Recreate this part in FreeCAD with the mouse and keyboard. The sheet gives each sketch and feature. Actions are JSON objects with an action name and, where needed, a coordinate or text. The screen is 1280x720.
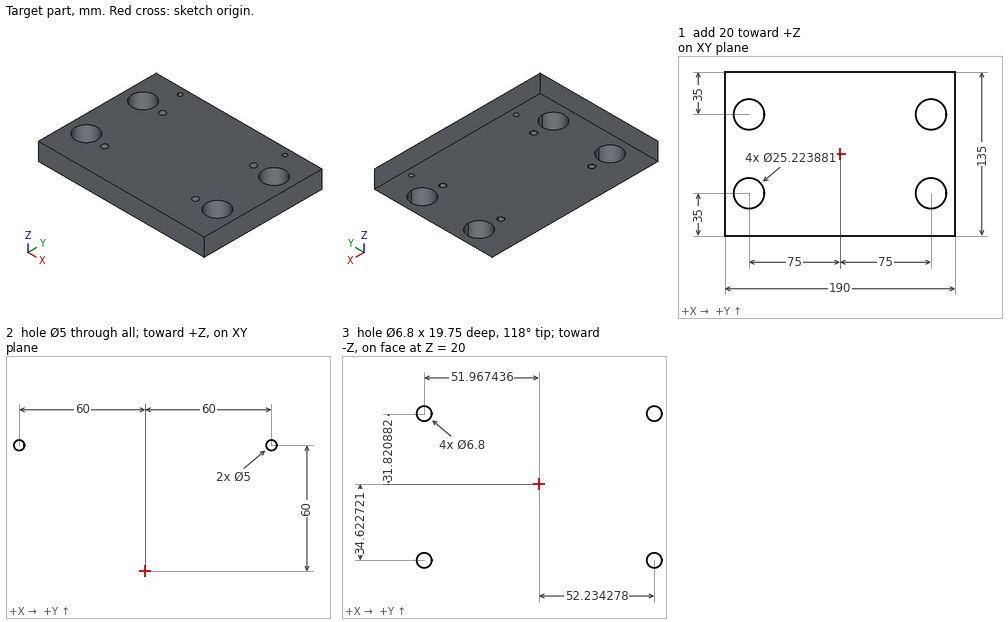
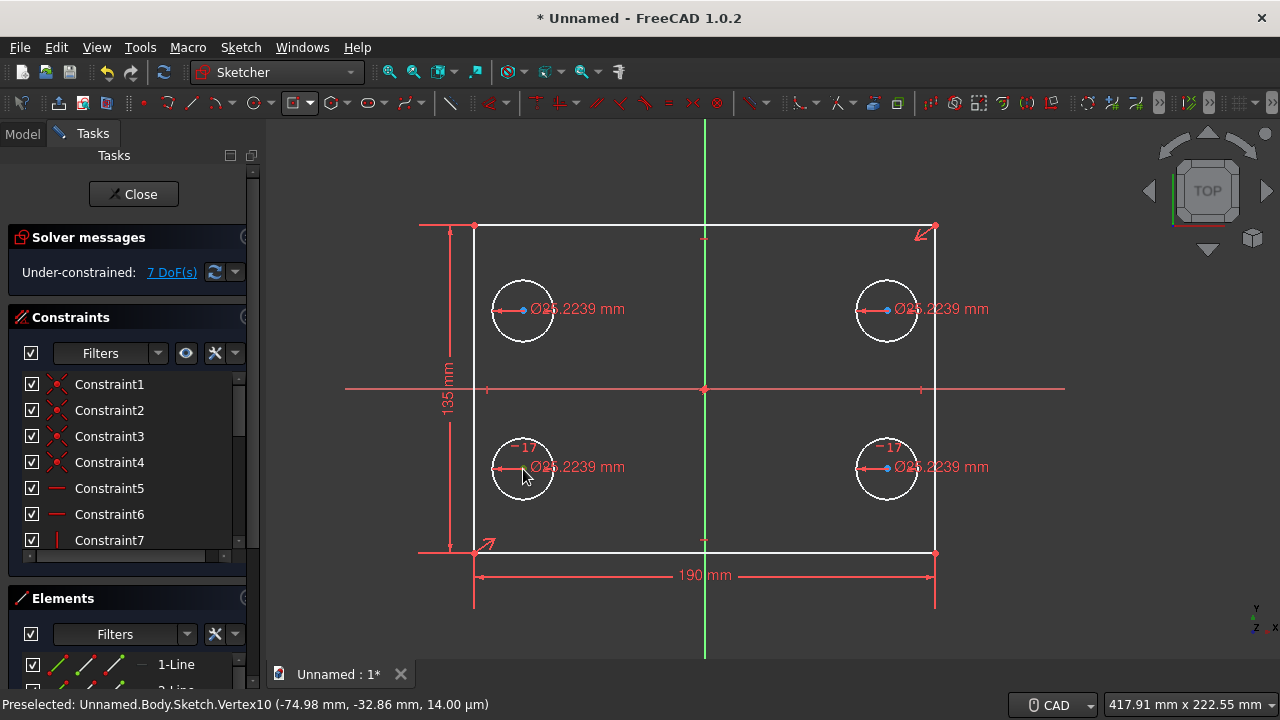
{"action": "left_click", "coordinate": [523, 311]}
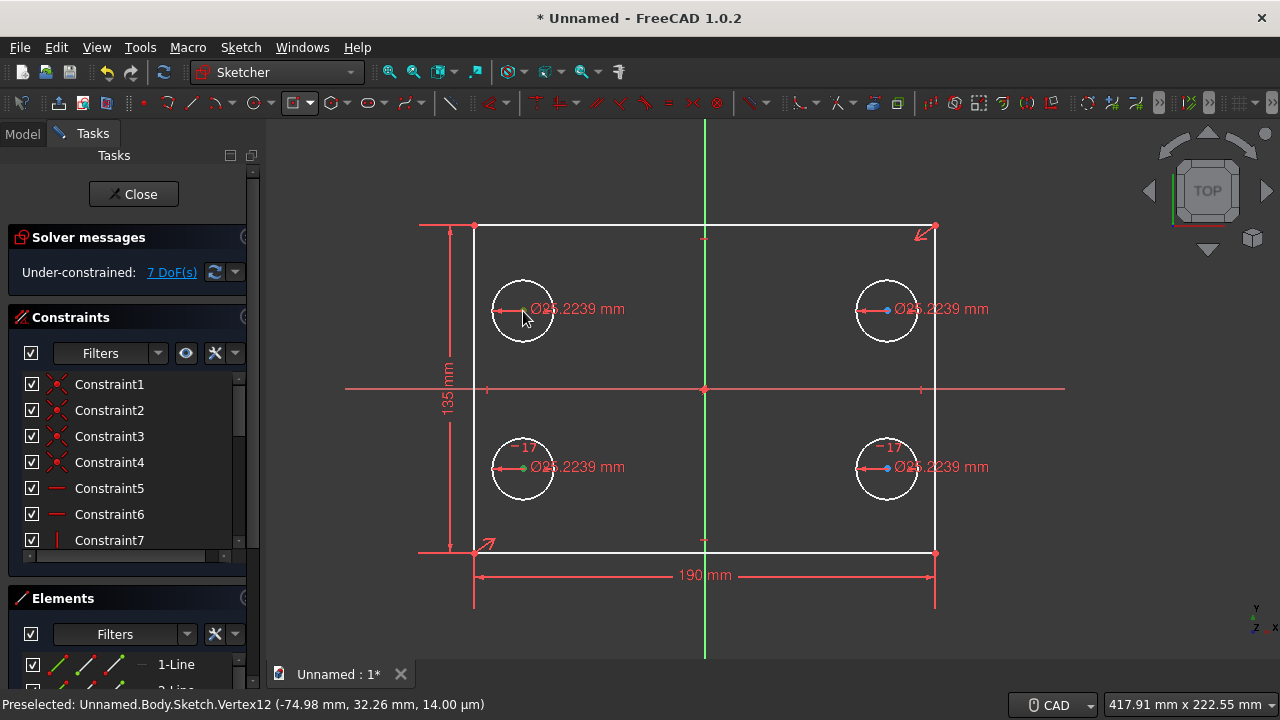
{"action": "left_click", "coordinate": [578, 104]}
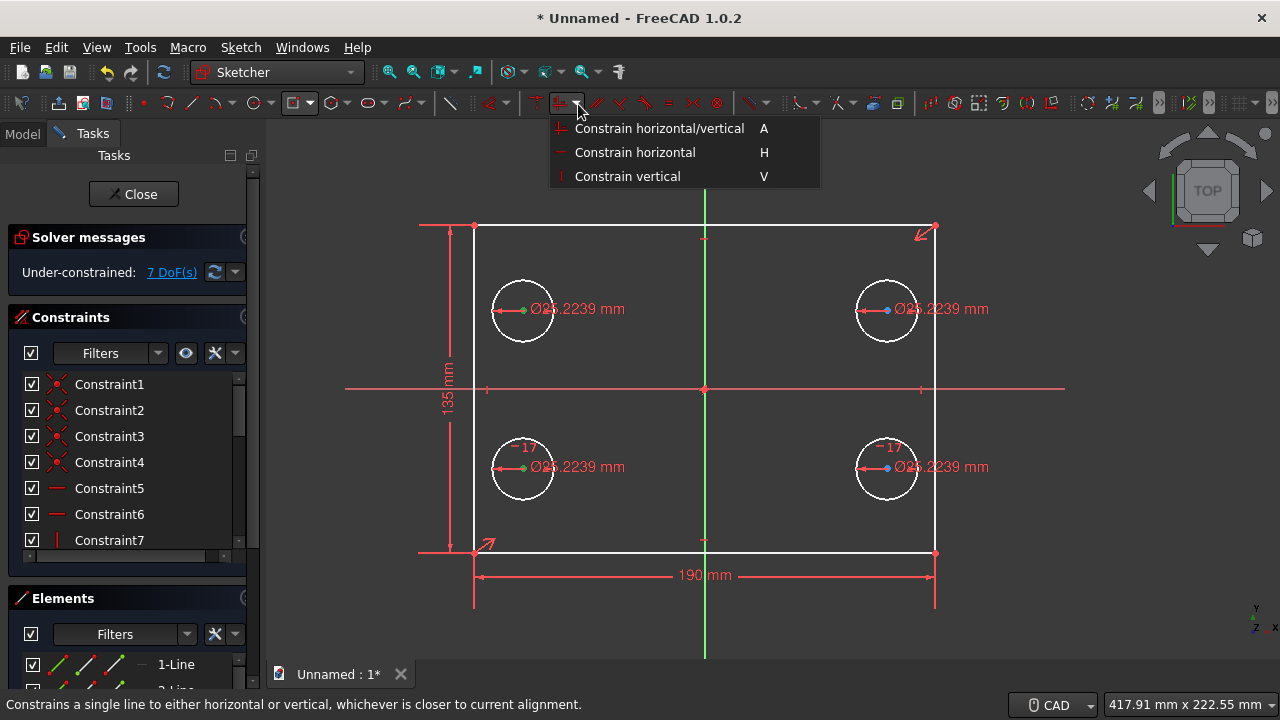
{"action": "left_click", "coordinate": [685, 176]}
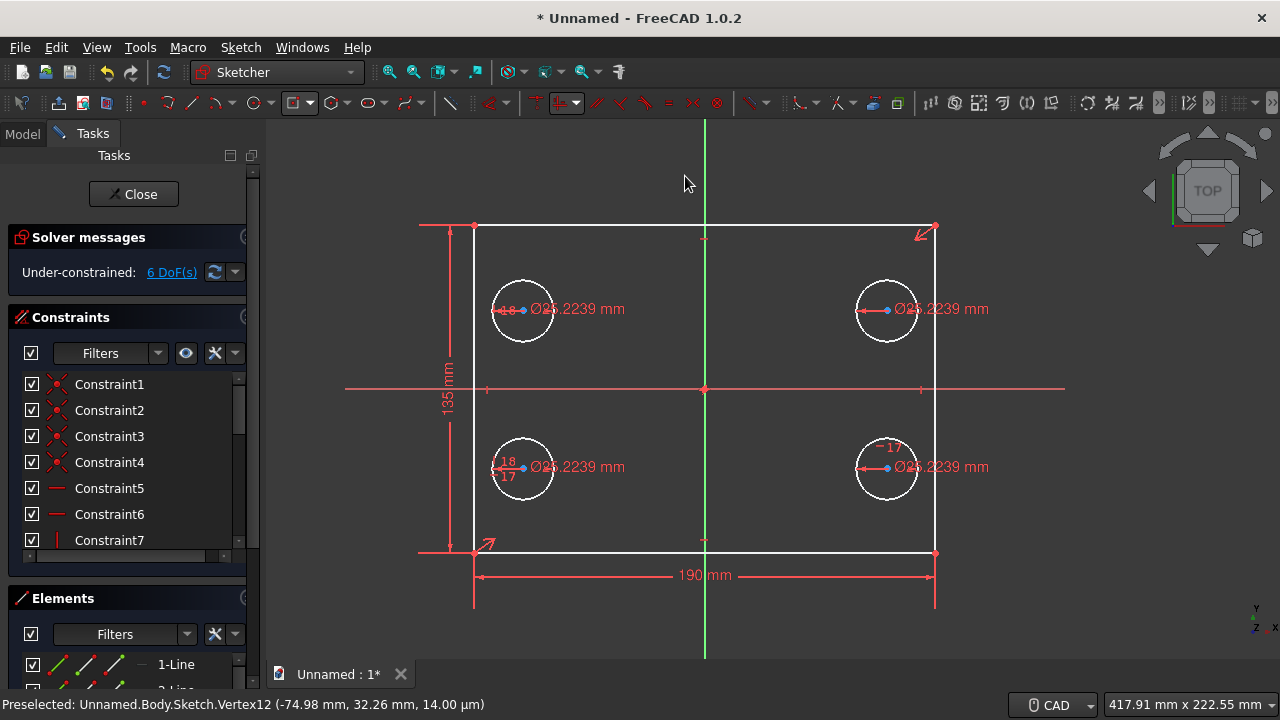
{"action": "left_click", "coordinate": [887, 469]}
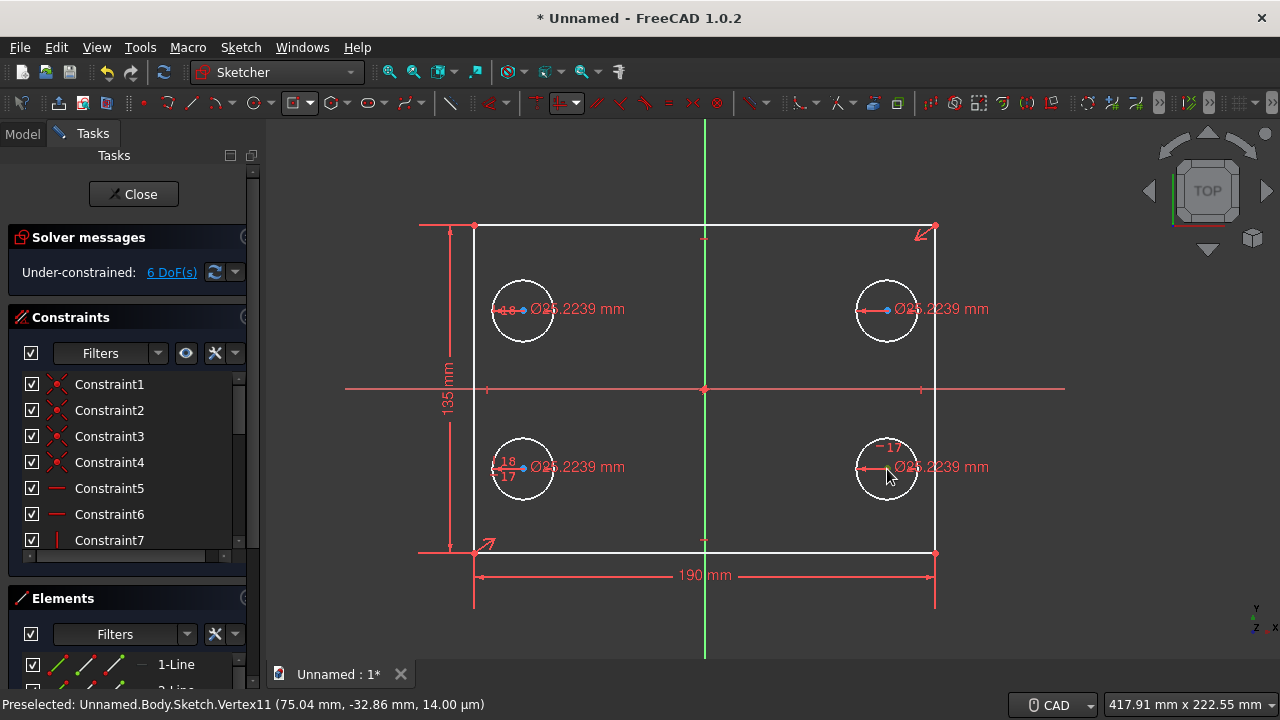
{"action": "left_click", "coordinate": [887, 311]}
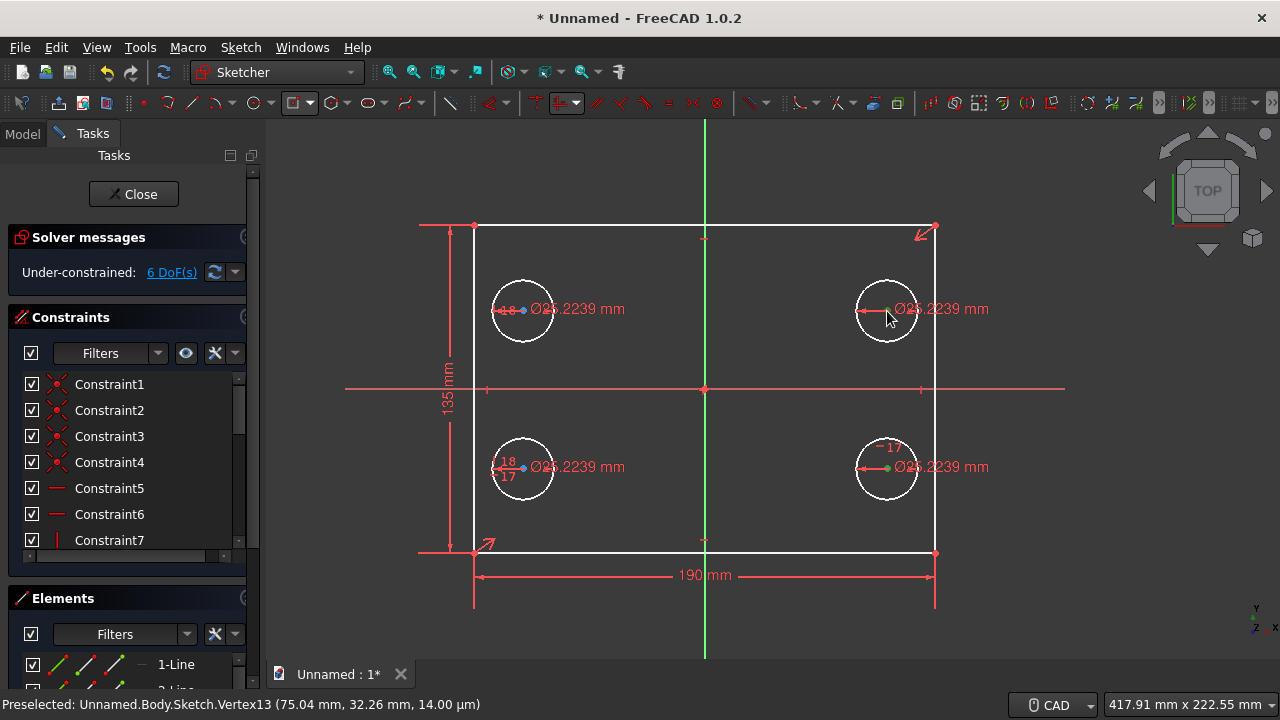
{"action": "left_click", "coordinate": [578, 104]}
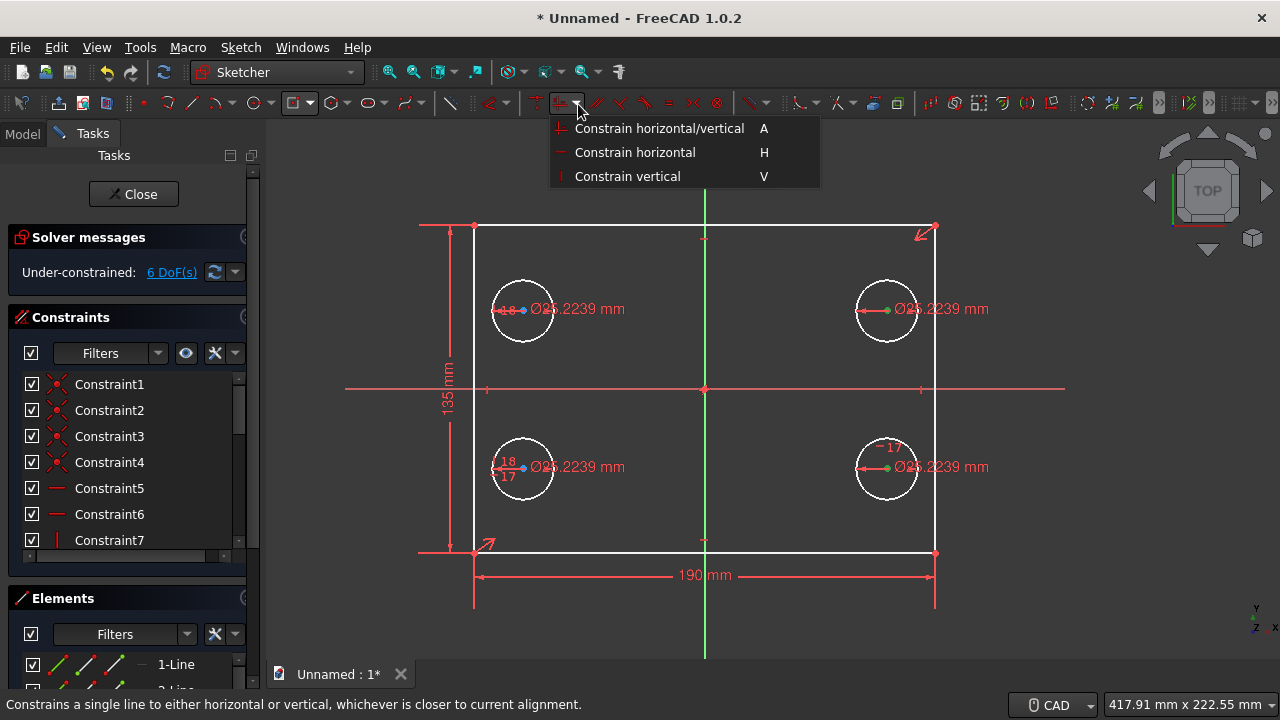
{"action": "left_click", "coordinate": [685, 176]}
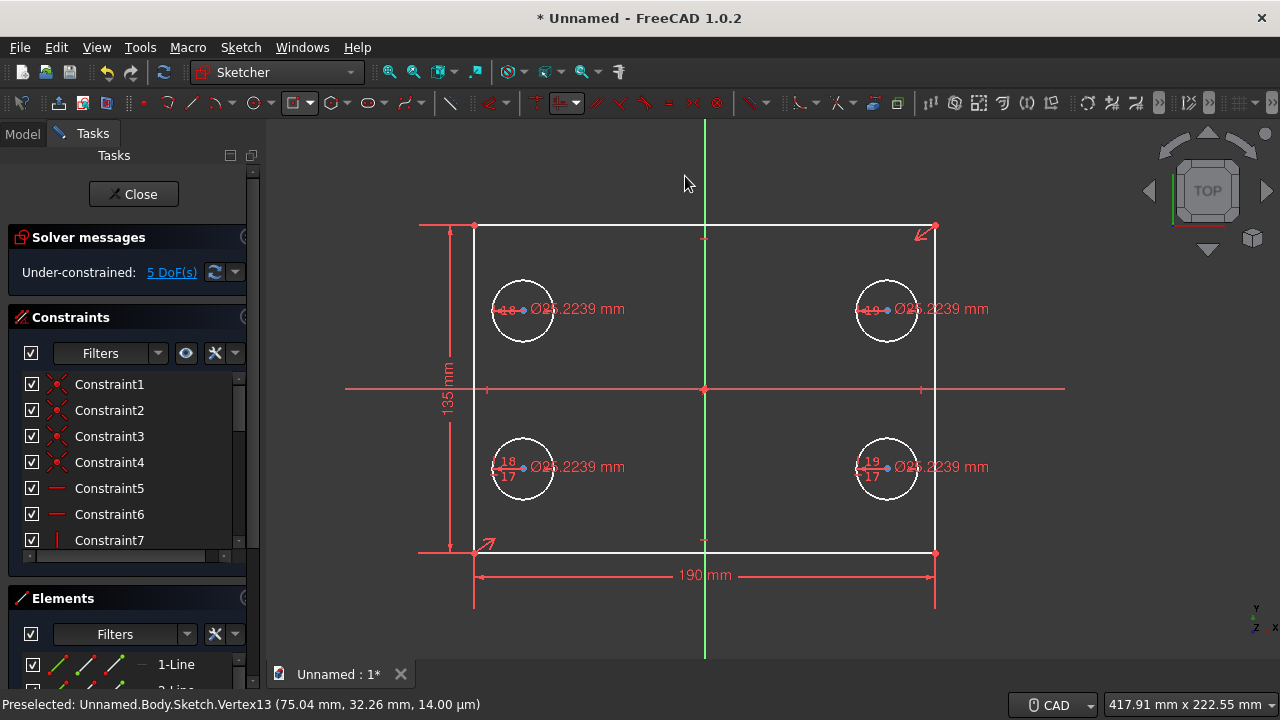
{"action": "left_click", "coordinate": [523, 311]}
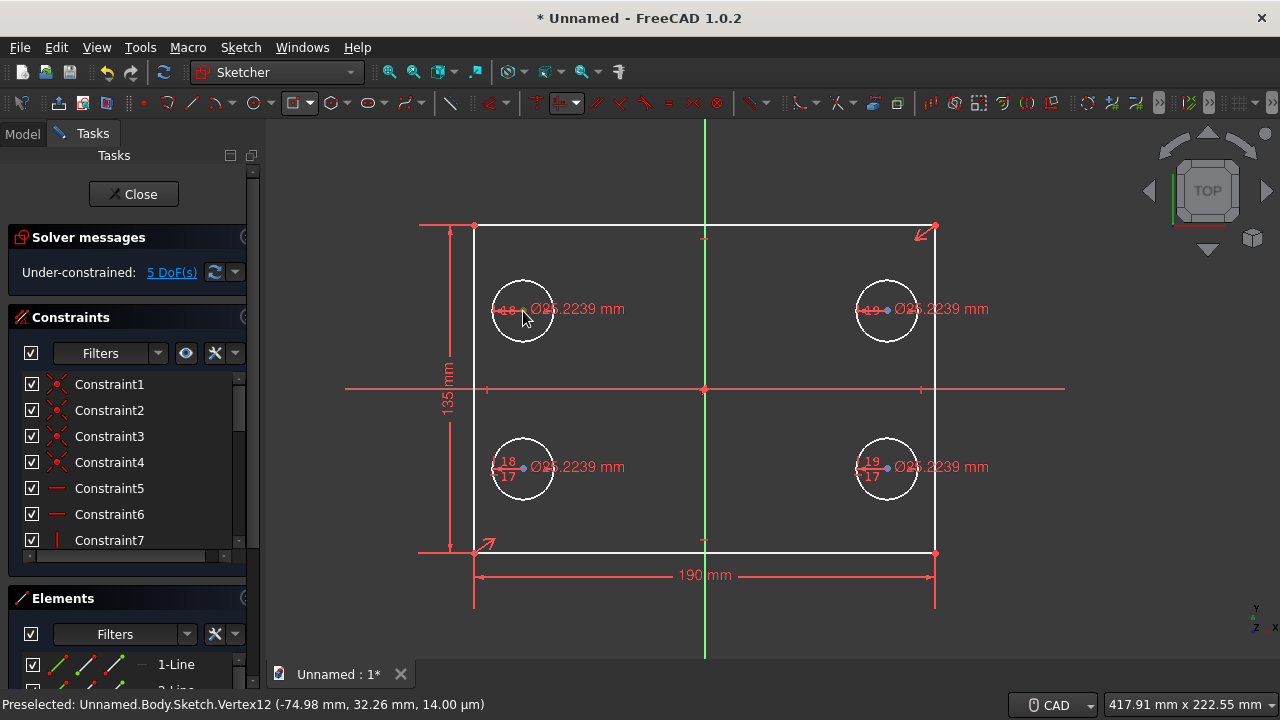
{"action": "left_click", "coordinate": [887, 311]}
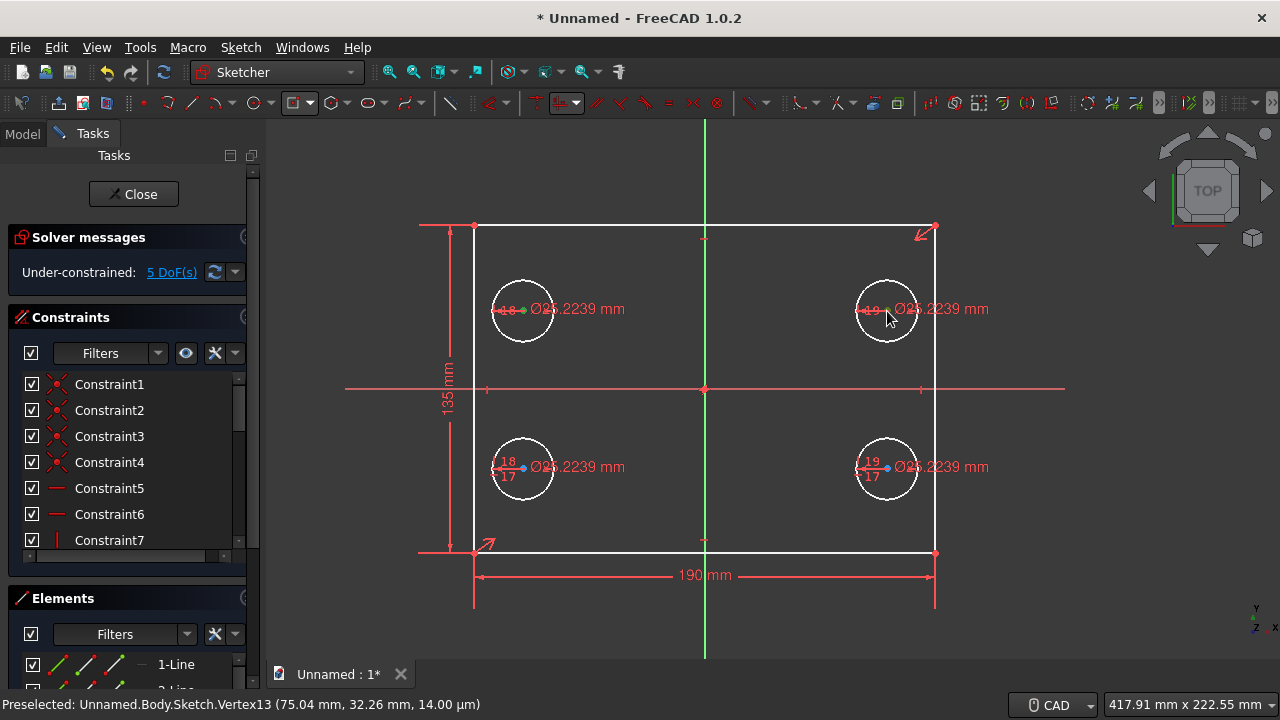
{"action": "left_click", "coordinate": [578, 104]}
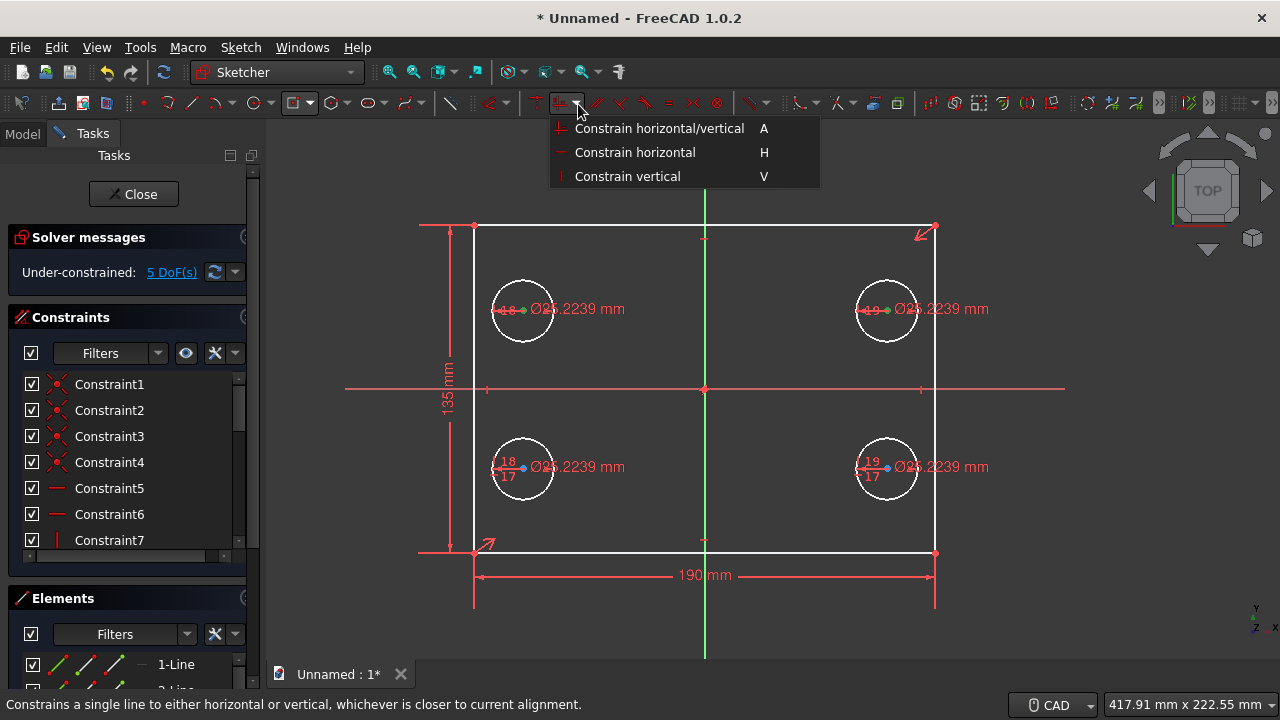
{"action": "left_click", "coordinate": [685, 152]}